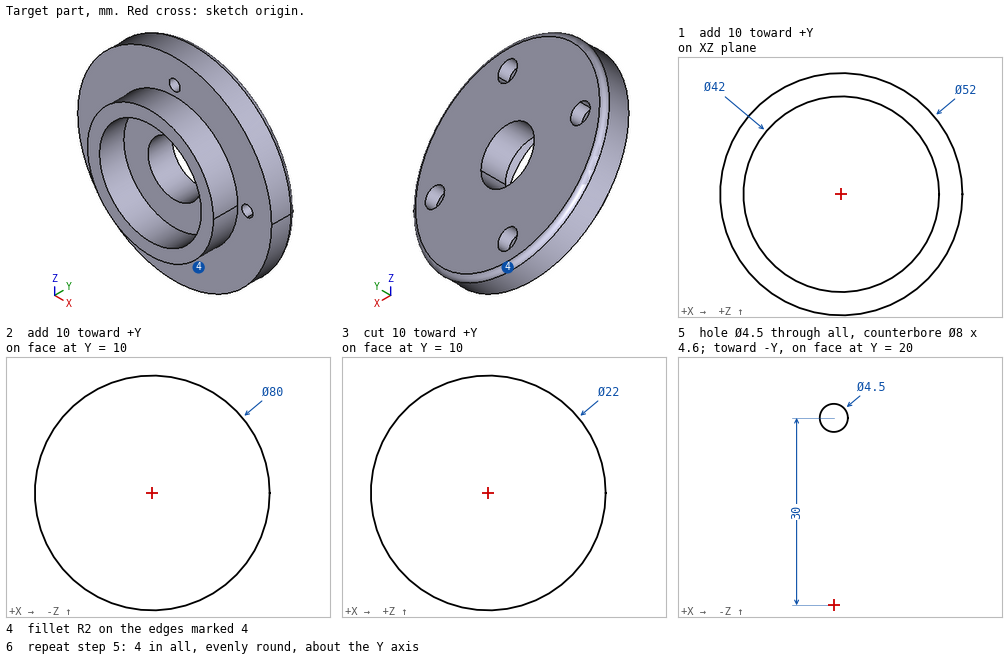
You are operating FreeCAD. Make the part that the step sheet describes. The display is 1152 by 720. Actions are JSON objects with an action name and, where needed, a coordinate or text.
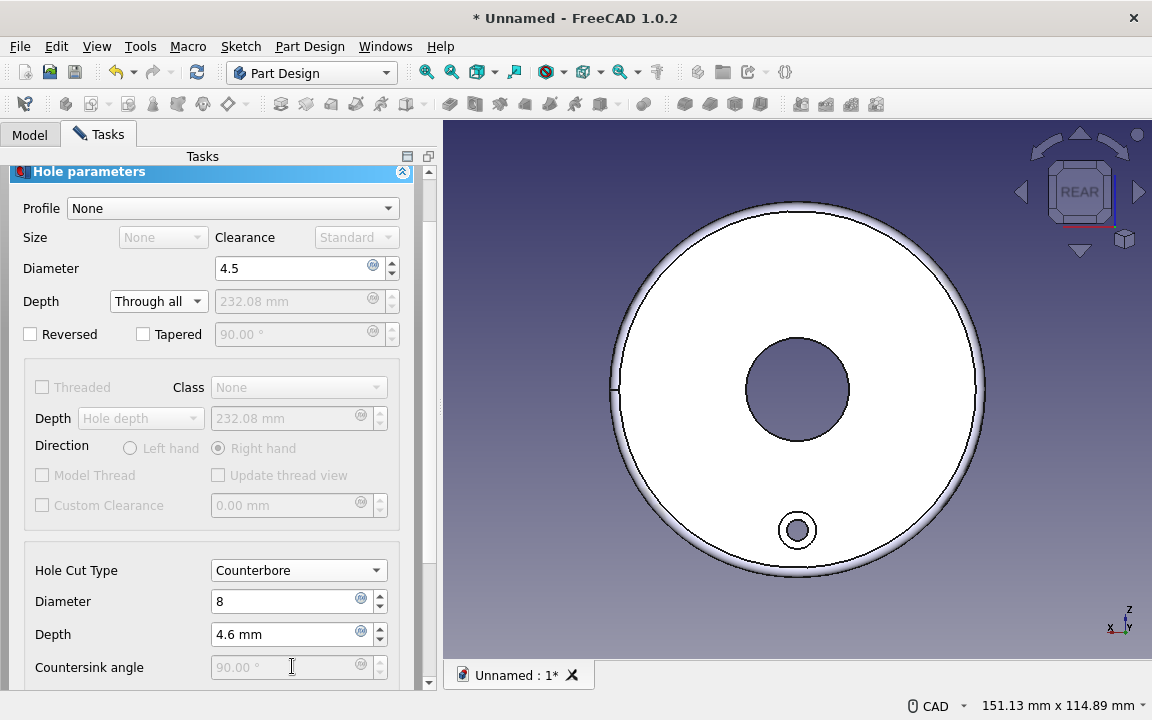
{"action": "scroll", "coordinate": [429, 428], "scroll_direction": "up", "scroll_amount": 2}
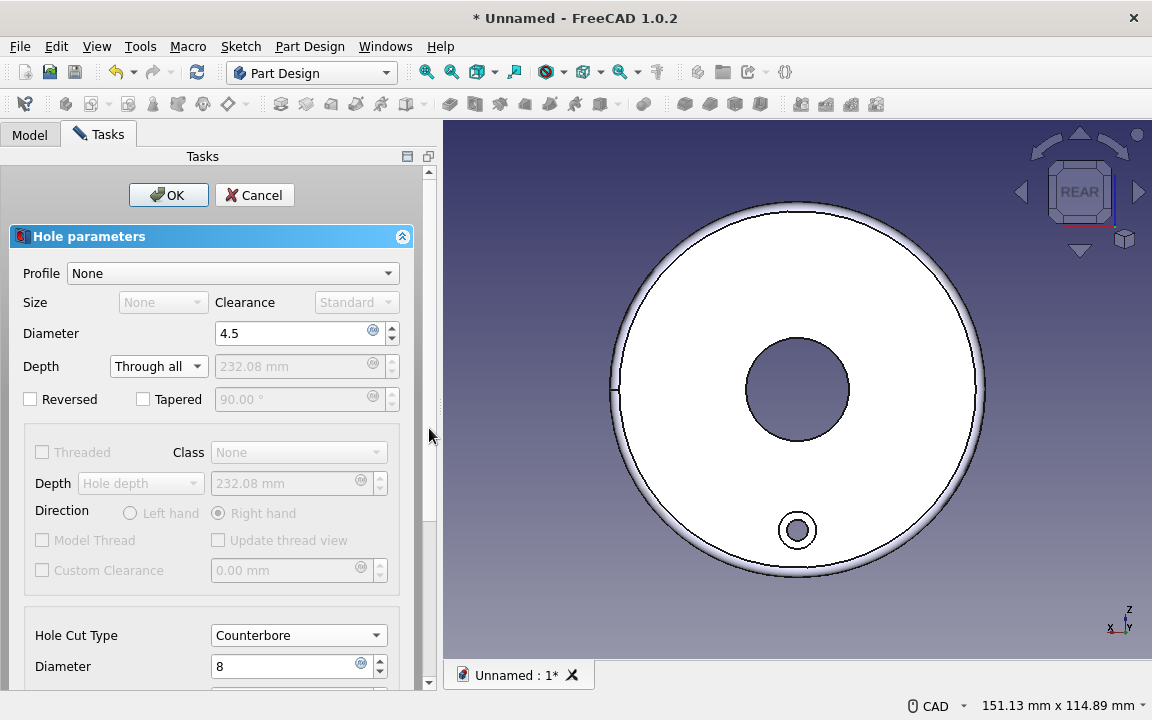
{"action": "left_click", "coordinate": [169, 195]}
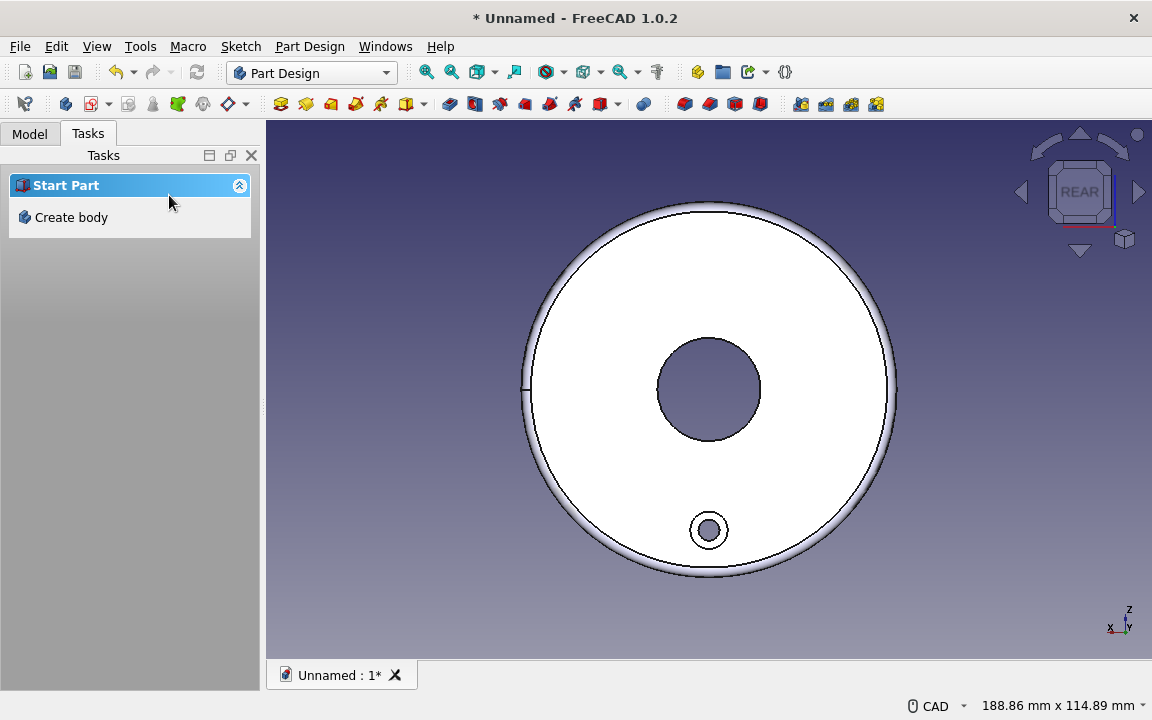
{"action": "left_click", "coordinate": [30, 134]}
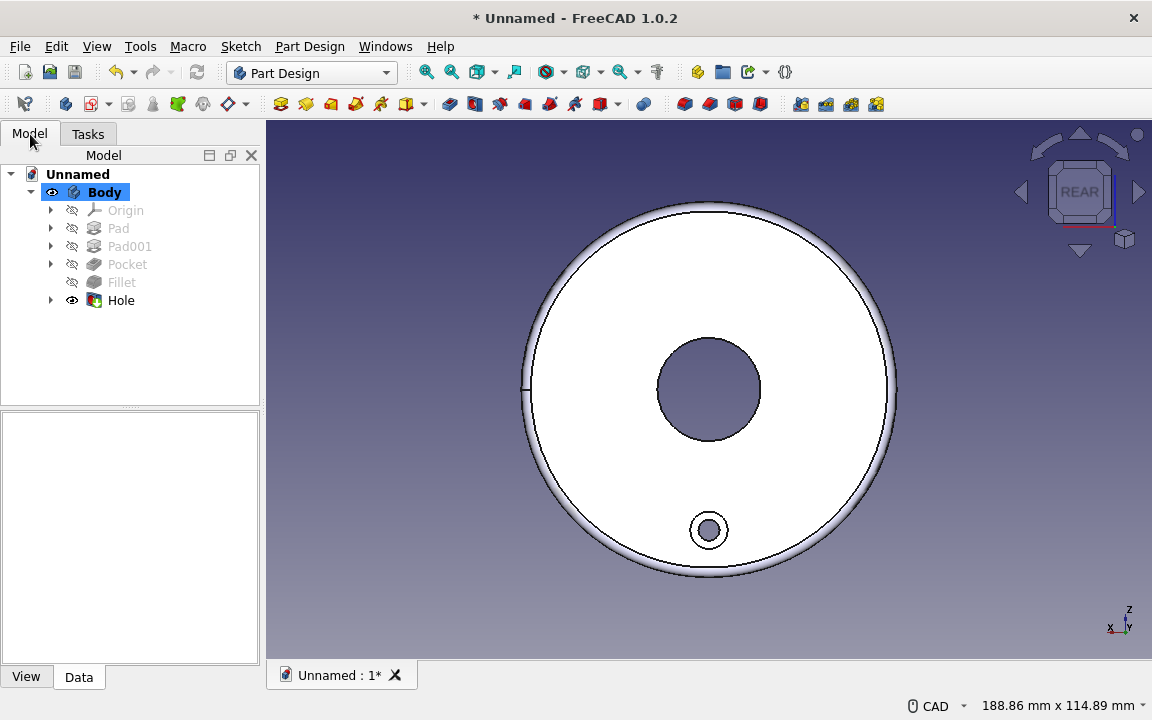
{"action": "left_click", "coordinate": [117, 300]}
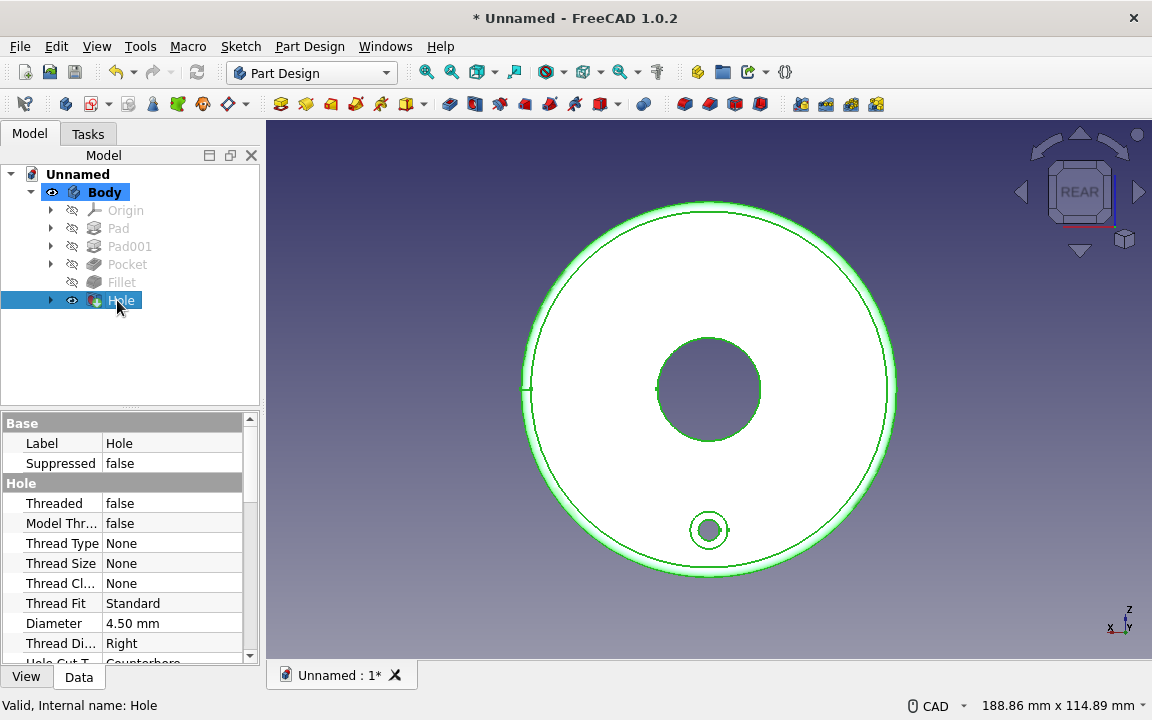
{"action": "left_click", "coordinate": [851, 104]}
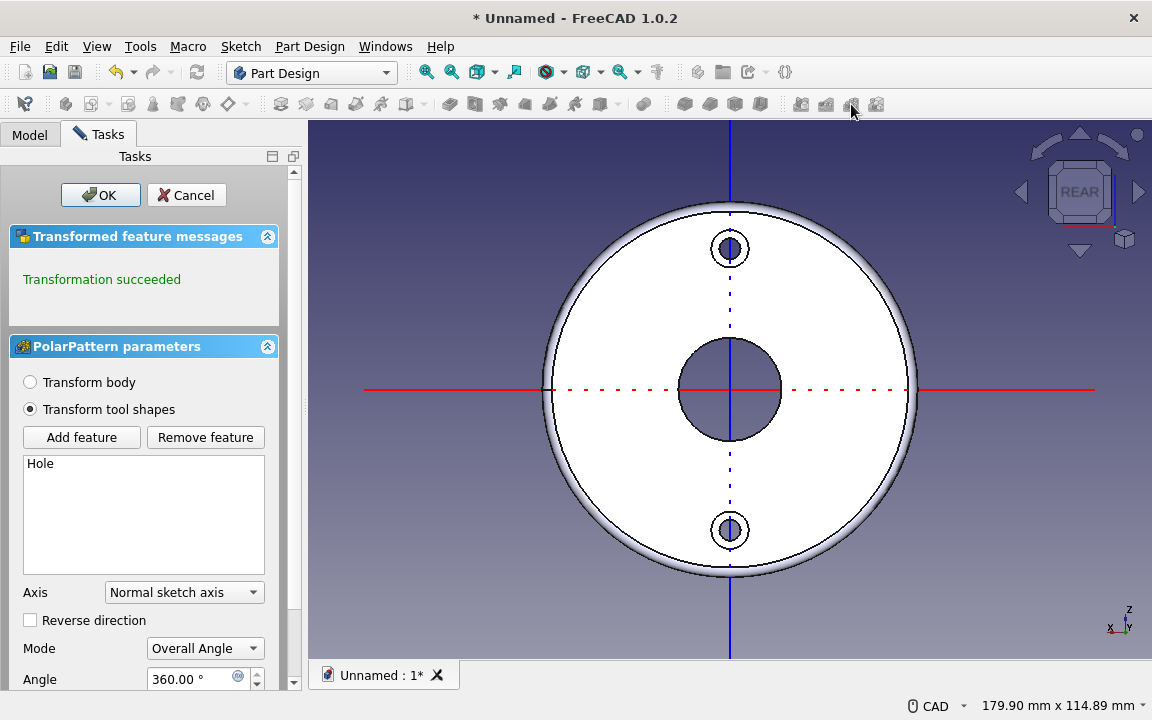
{"action": "left_click", "coordinate": [185, 592]}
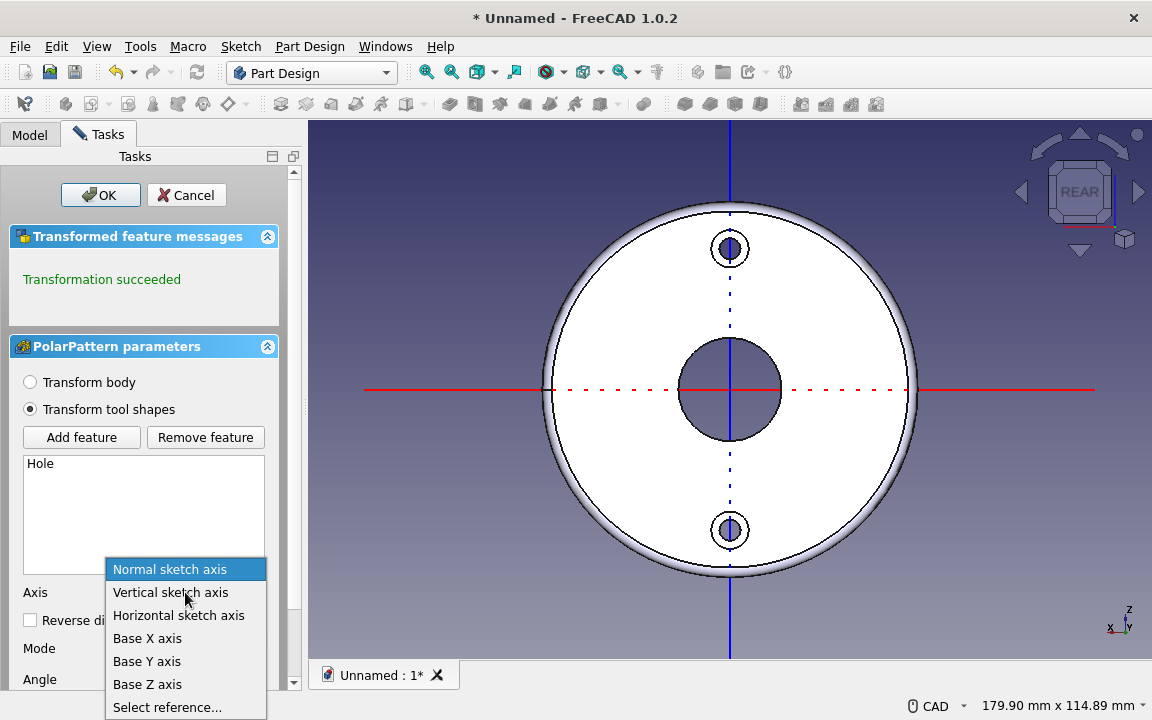
{"action": "left_click", "coordinate": [184, 662]}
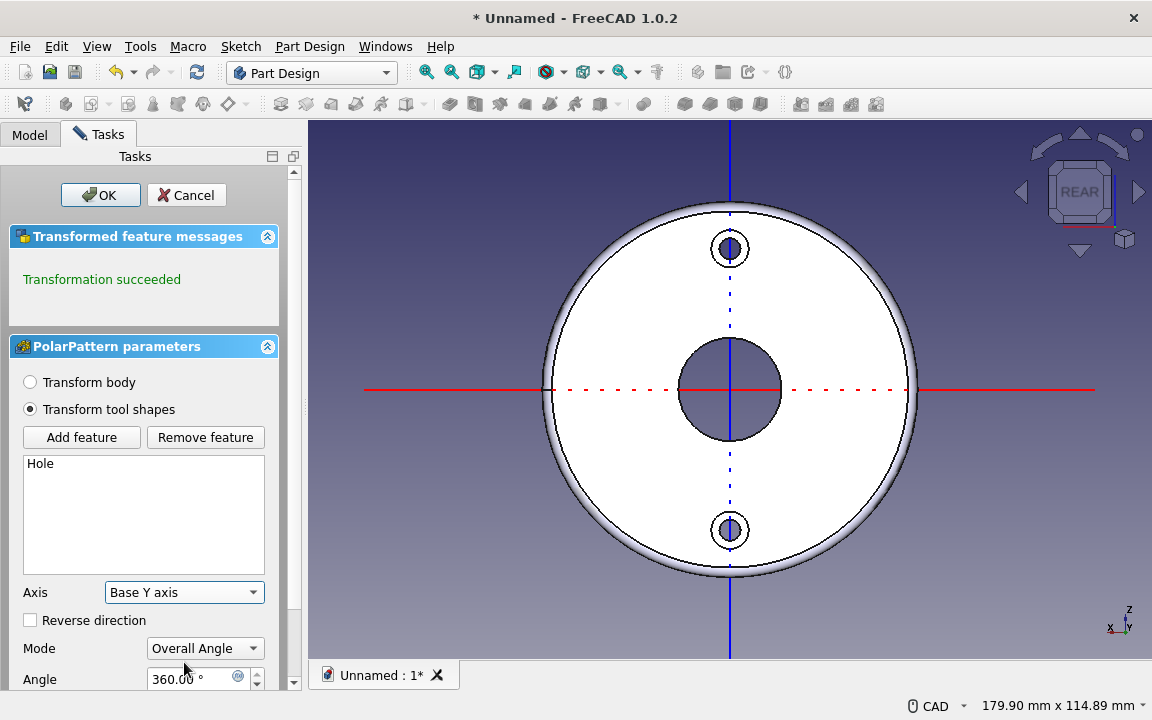
{"action": "scroll", "coordinate": [294, 428], "scroll_direction": "down", "scroll_amount": 2}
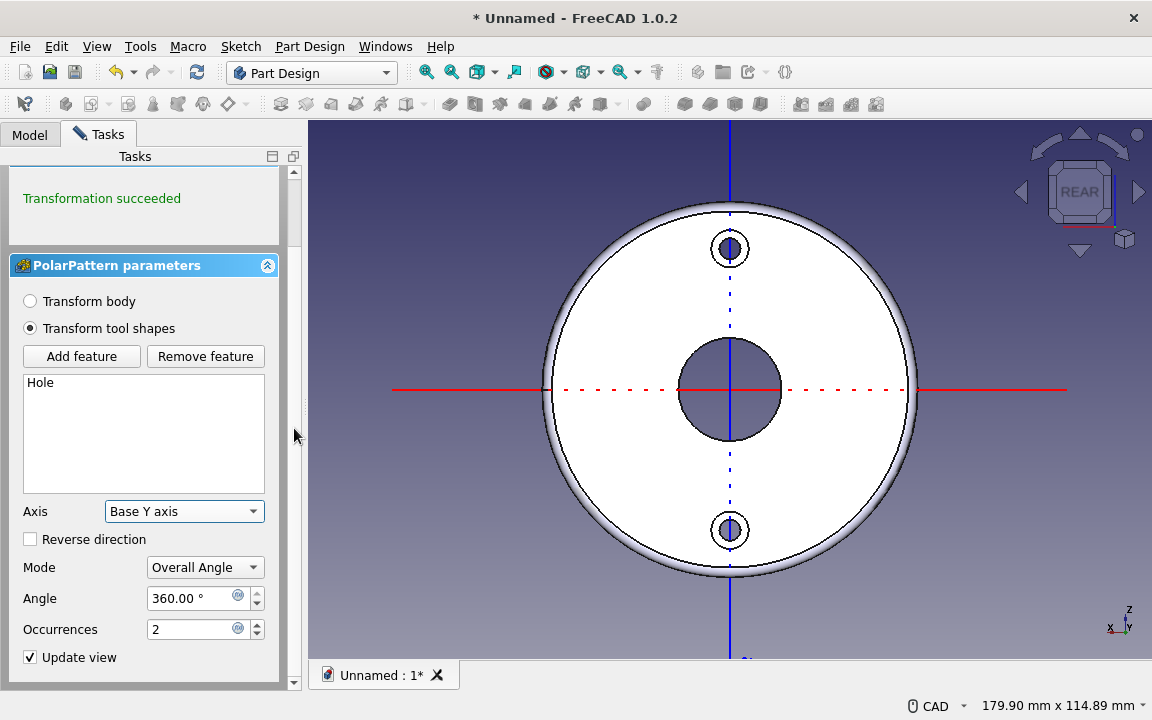
{"action": "triple_click", "coordinate": [199, 630]}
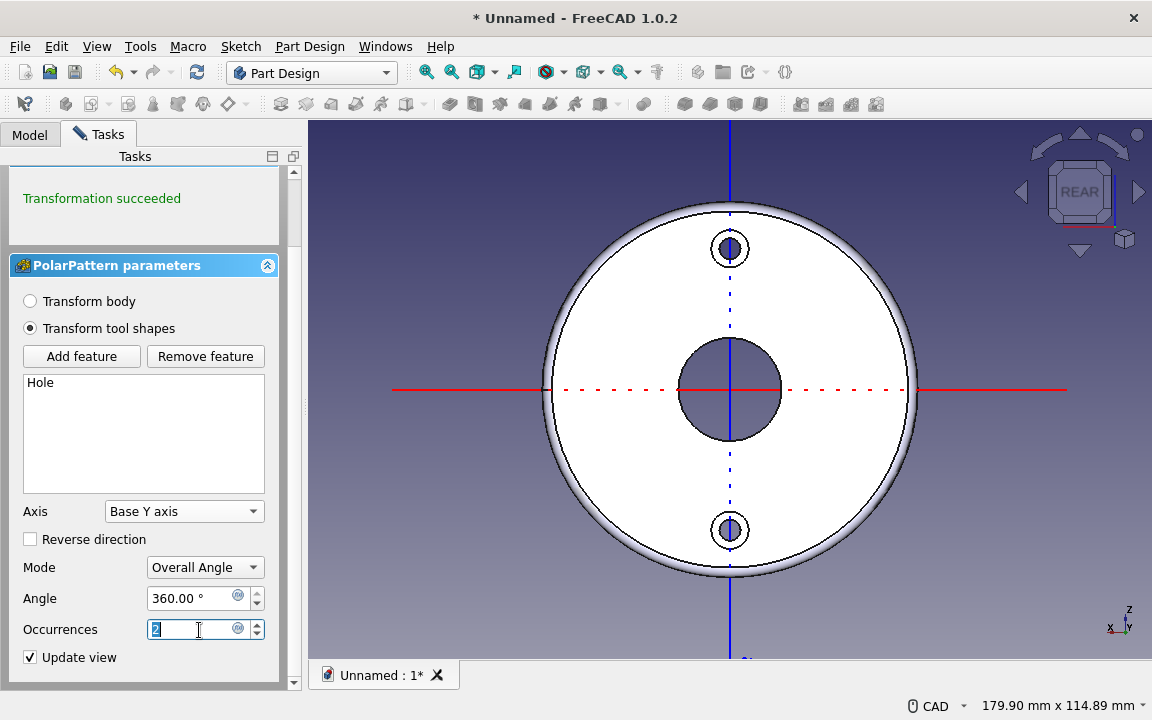
{"action": "type", "text": "4"}
{"action": "key", "text": "Tab"}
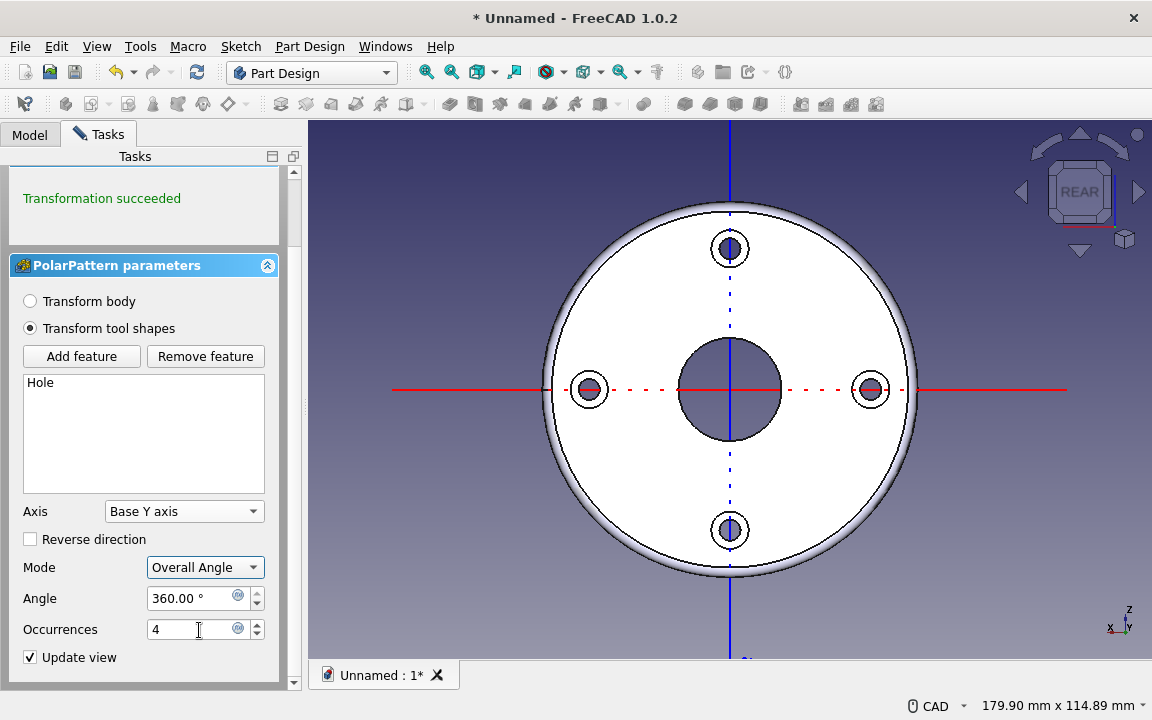
{"action": "scroll", "coordinate": [294, 428], "scroll_direction": "up", "scroll_amount": 3}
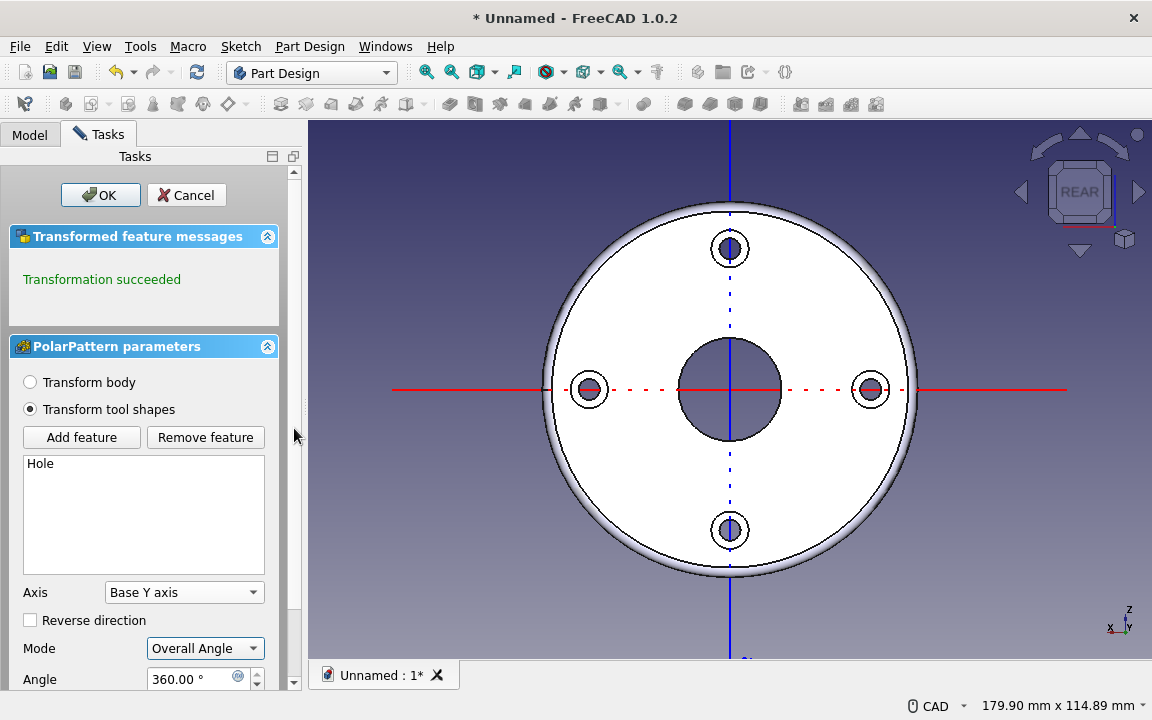
{"action": "left_click", "coordinate": [101, 195]}